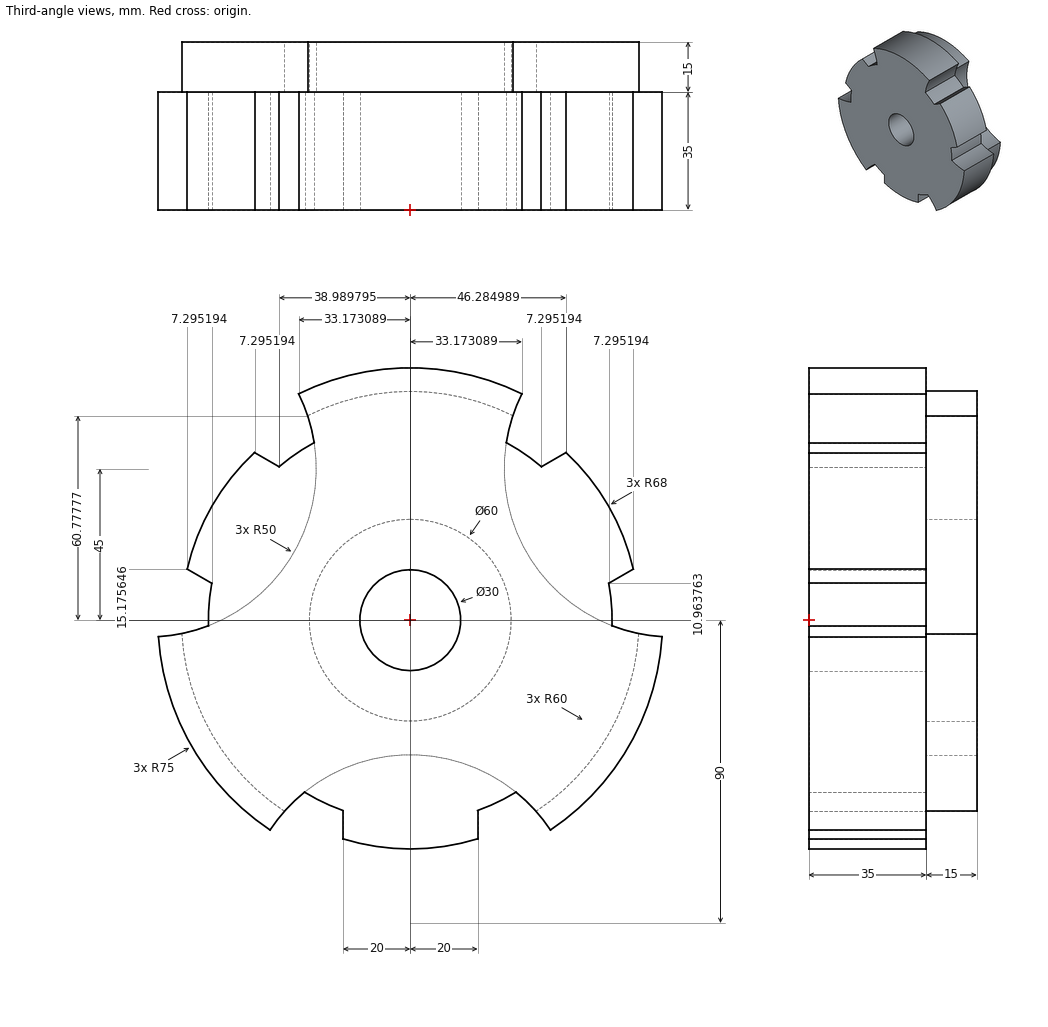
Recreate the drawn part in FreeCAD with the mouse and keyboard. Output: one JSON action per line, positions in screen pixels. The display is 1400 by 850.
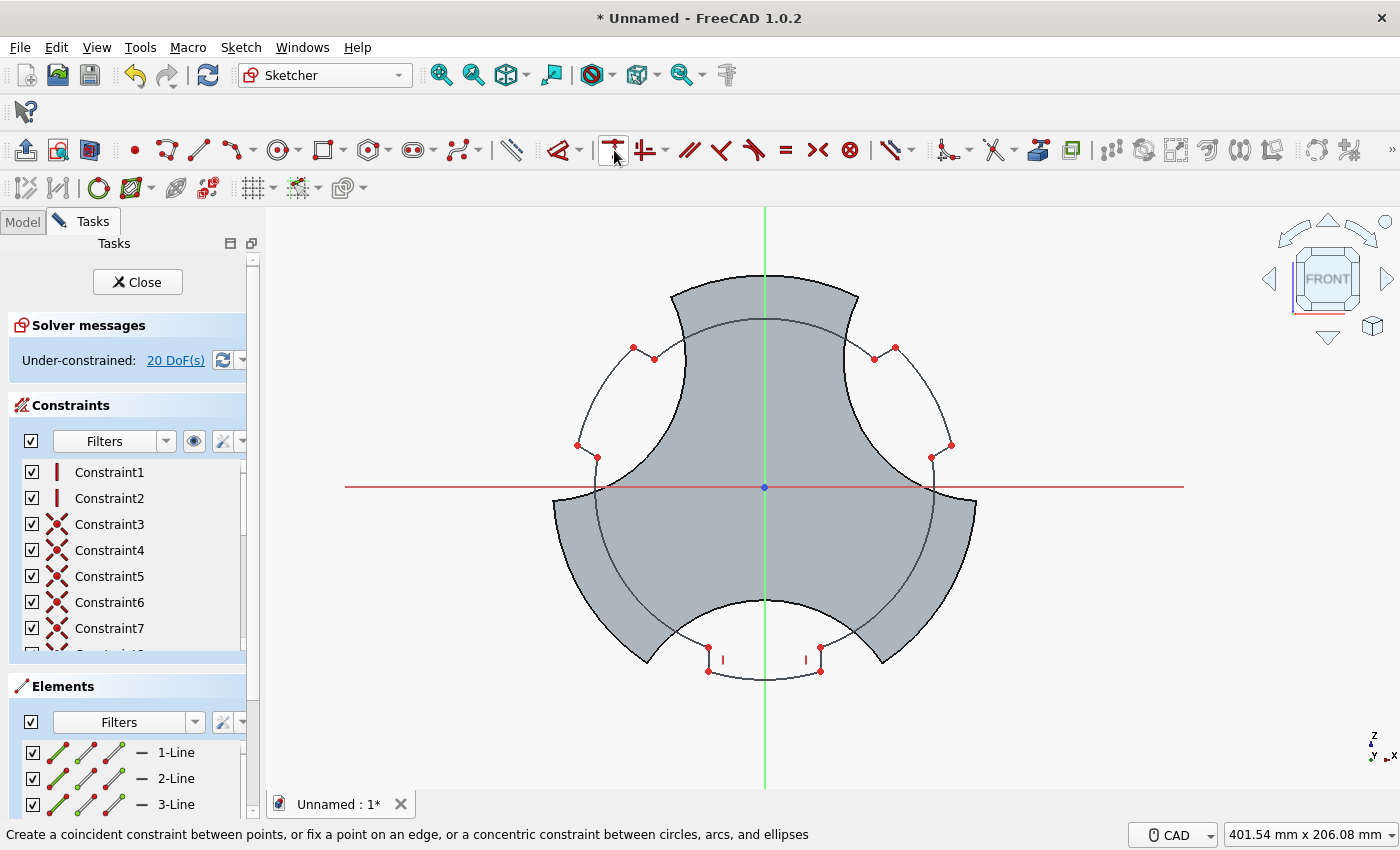
{"action": "left_click", "coordinate": [882, 610]}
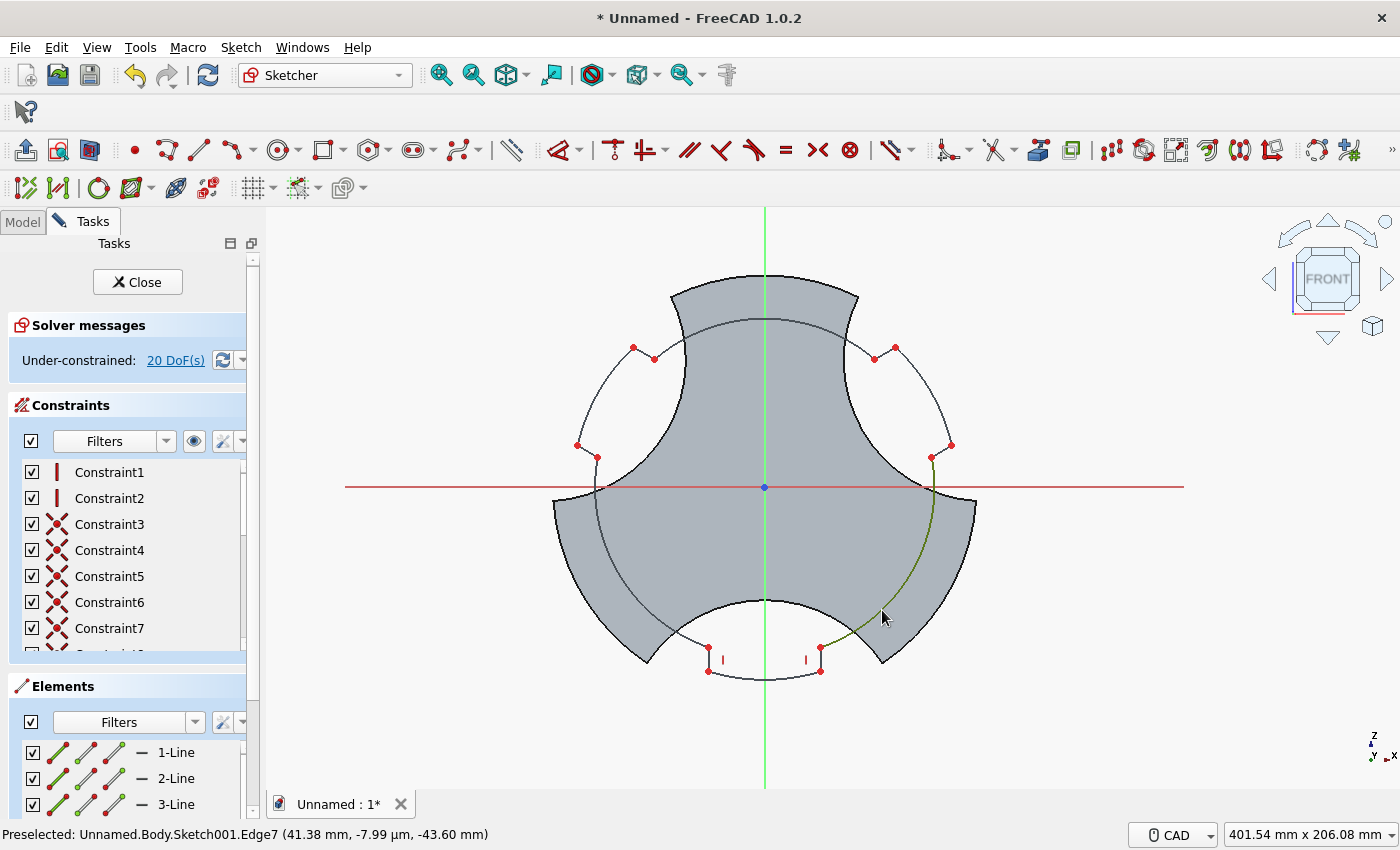
{"action": "left_click", "coordinate": [742, 678]}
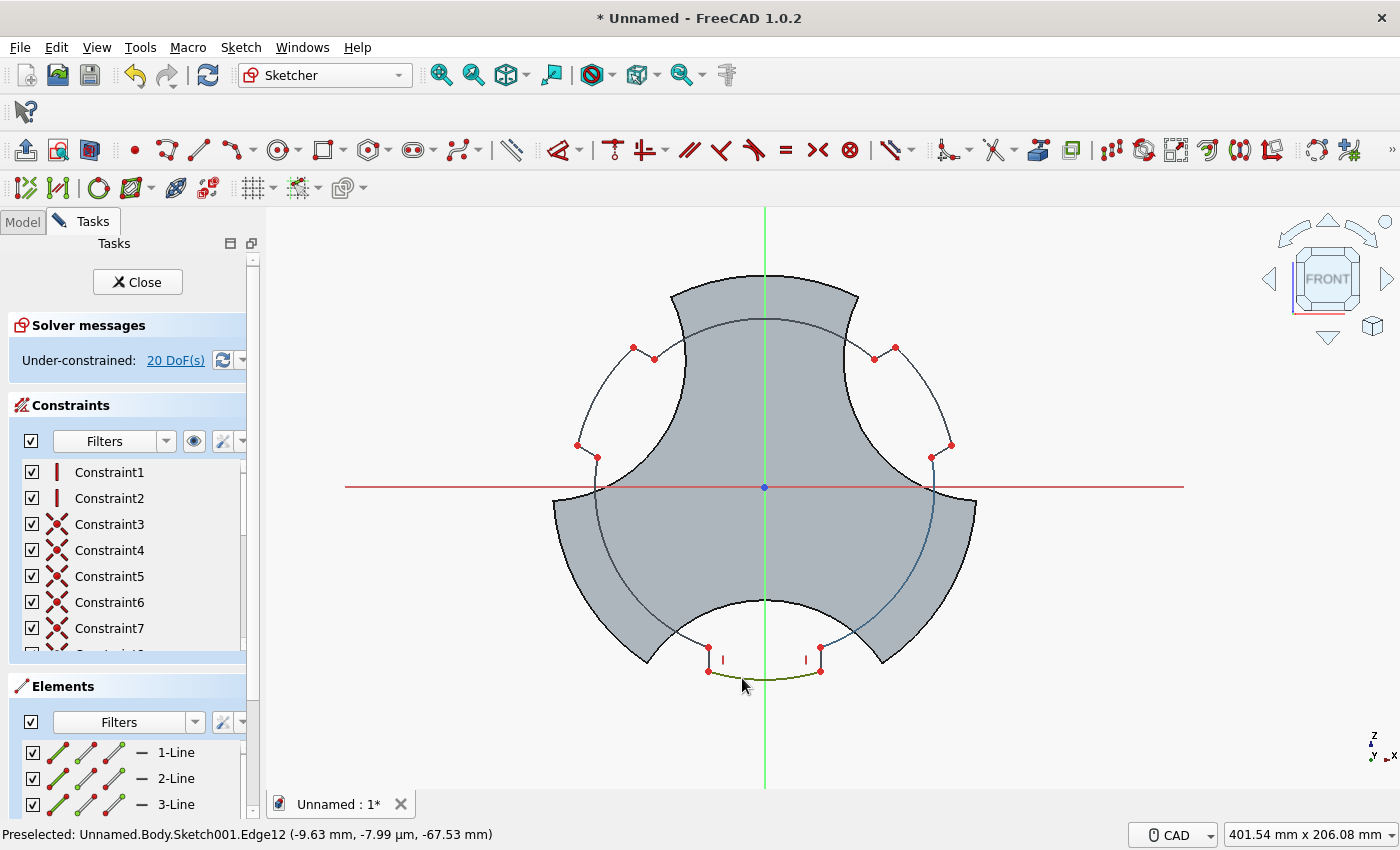
{"action": "left_click", "coordinate": [614, 150]}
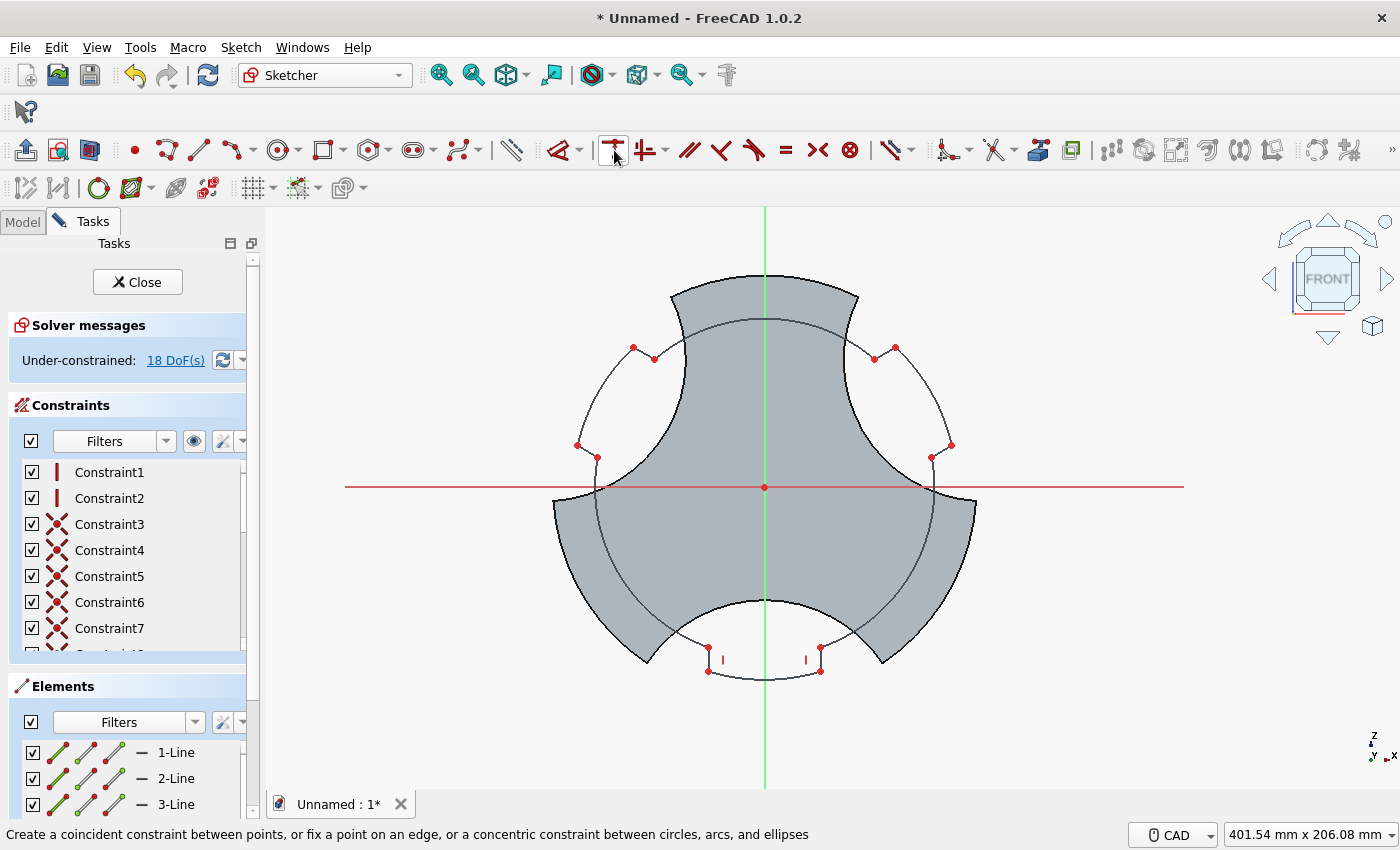
{"action": "left_click_drag", "start_coordinate": [755, 477], "coordinate": [775, 497]}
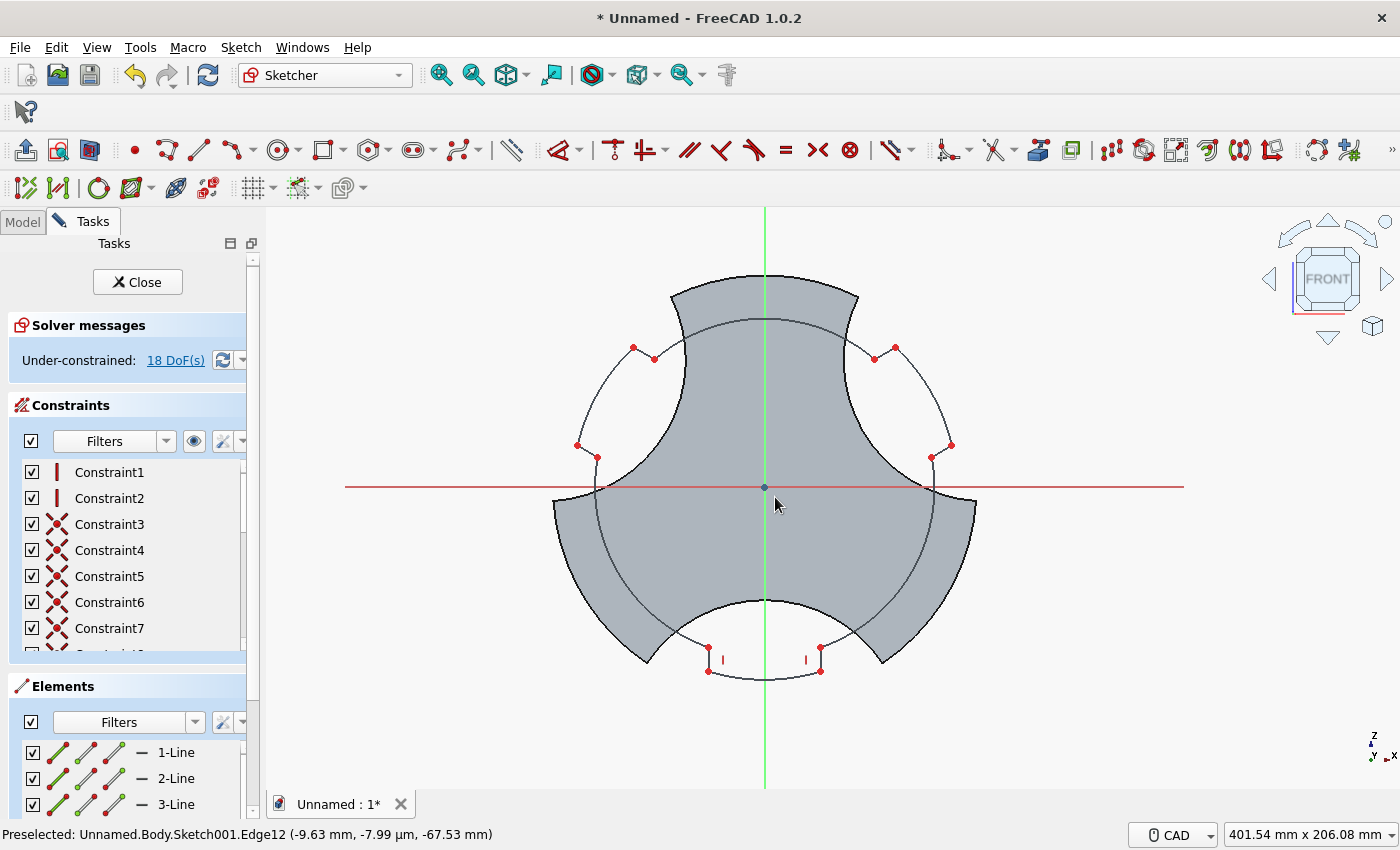
{"action": "left_click", "coordinate": [614, 150]}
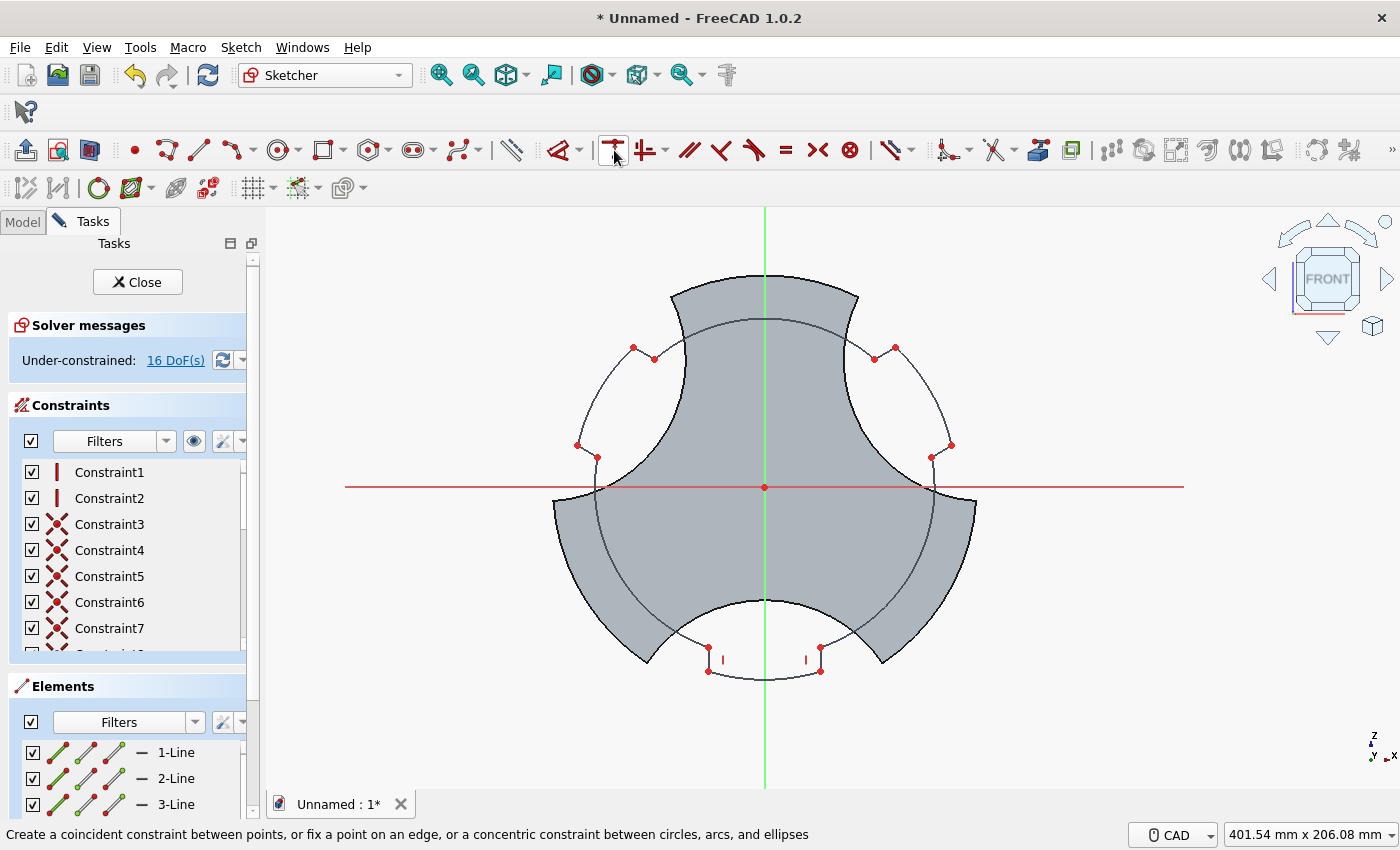
{"action": "left_click", "coordinate": [882, 610]}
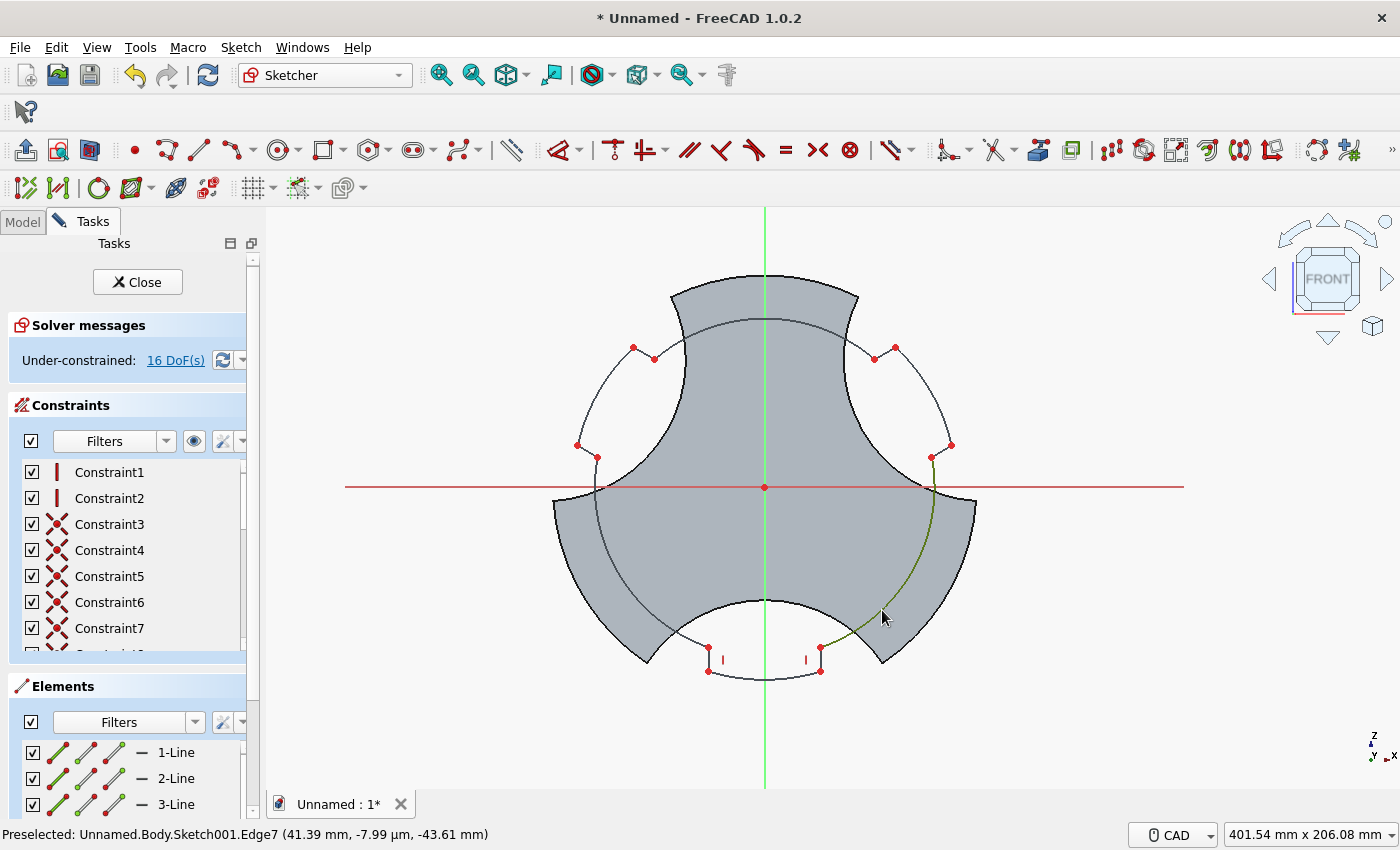
{"action": "left_click", "coordinate": [812, 325]}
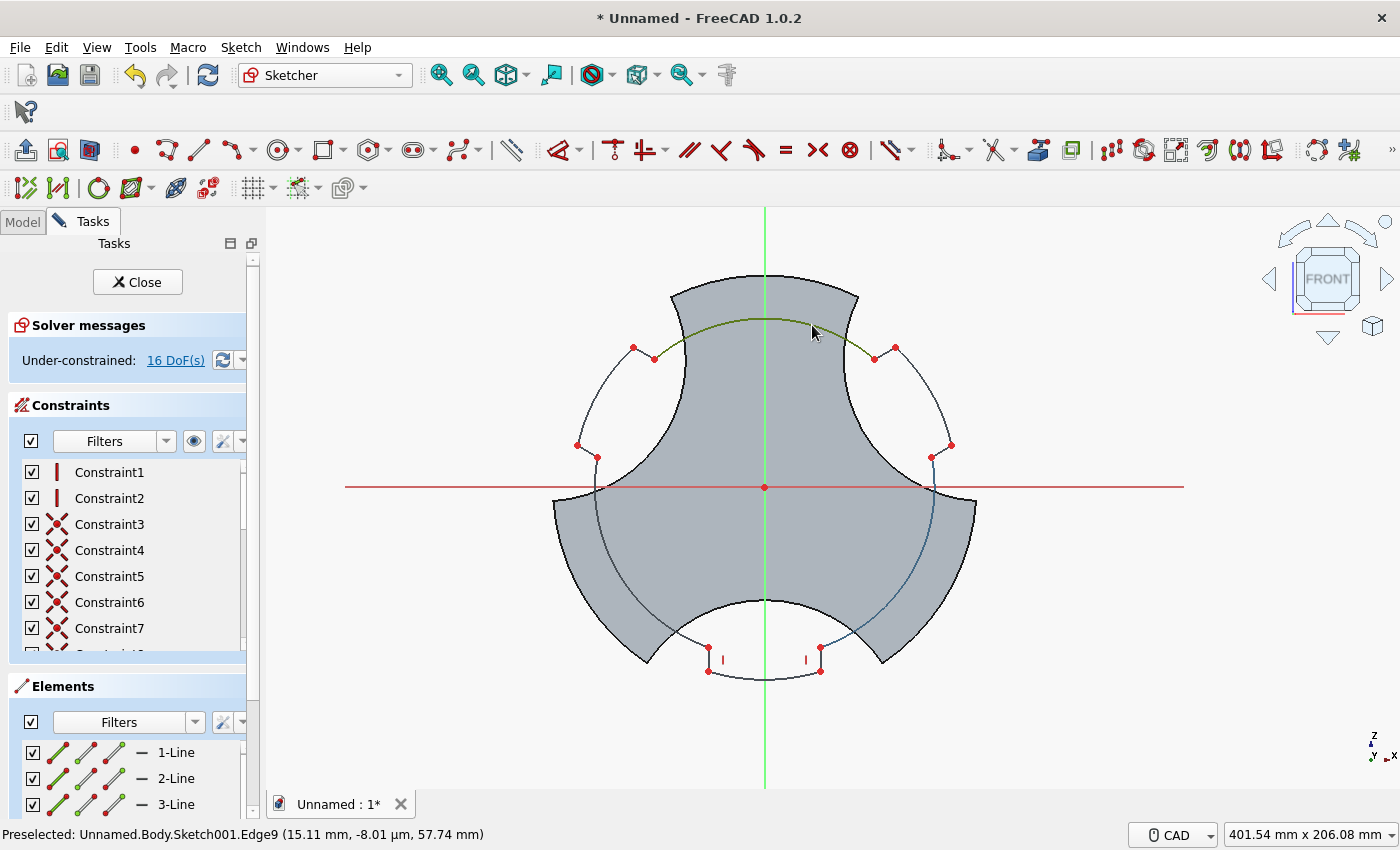
{"action": "left_click", "coordinate": [600, 529]}